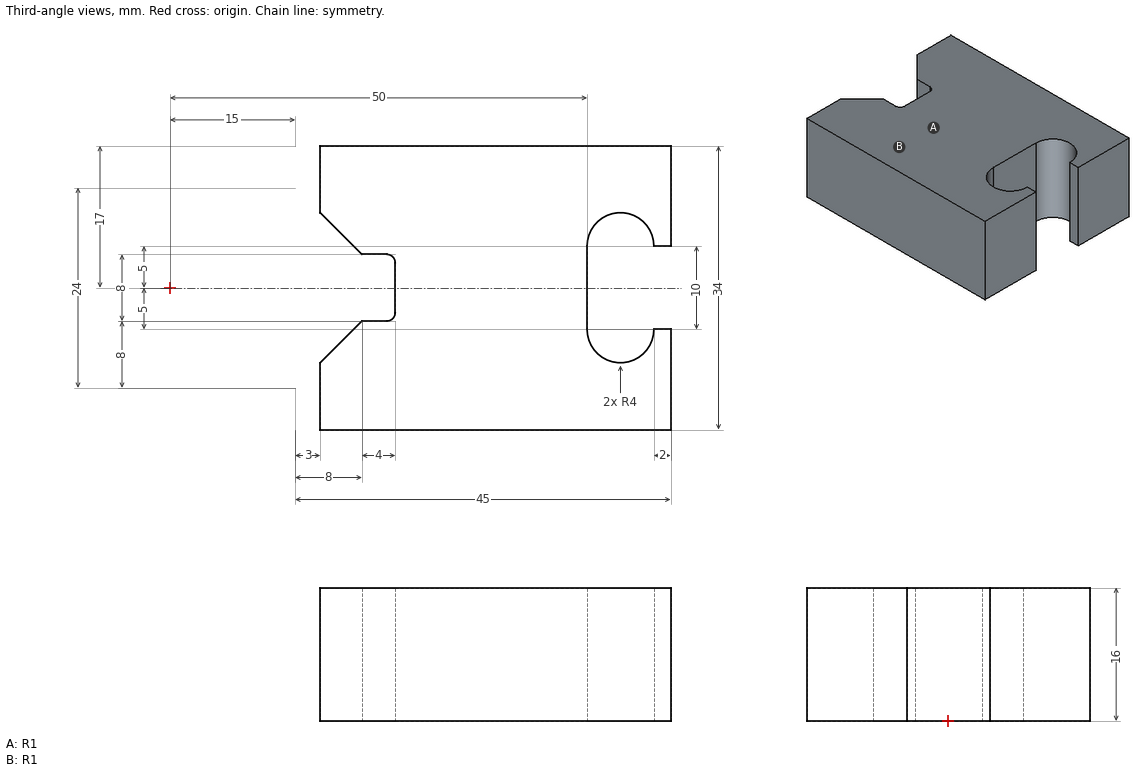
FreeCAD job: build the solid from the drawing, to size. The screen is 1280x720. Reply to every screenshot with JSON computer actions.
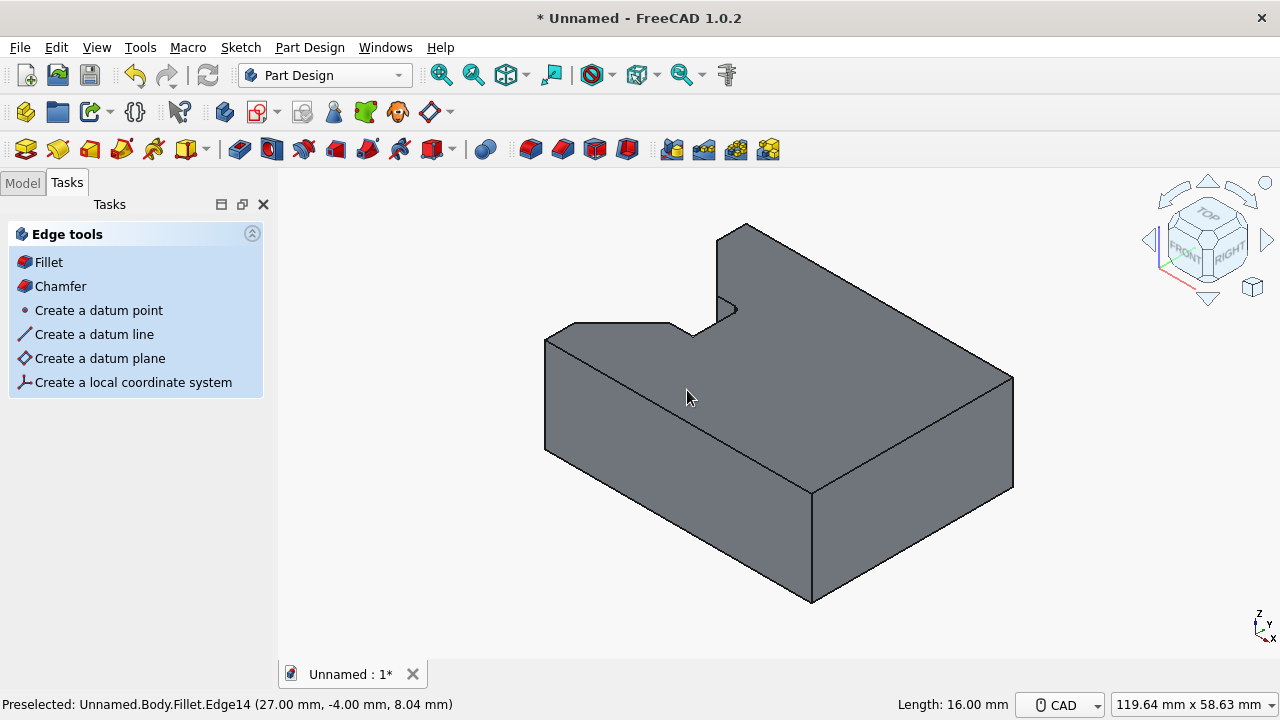
{"action": "left_click", "coordinate": [532, 150]}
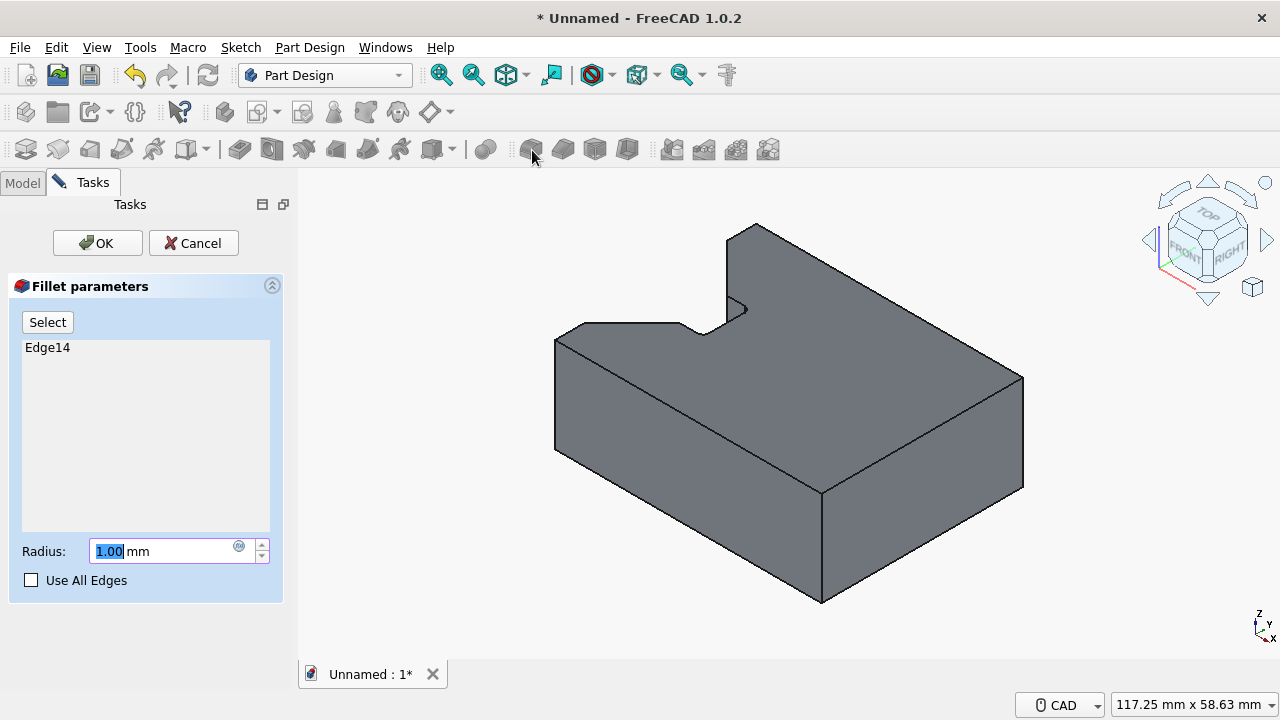
{"action": "type", "text": "1"}
{"action": "key", "text": "Tab"}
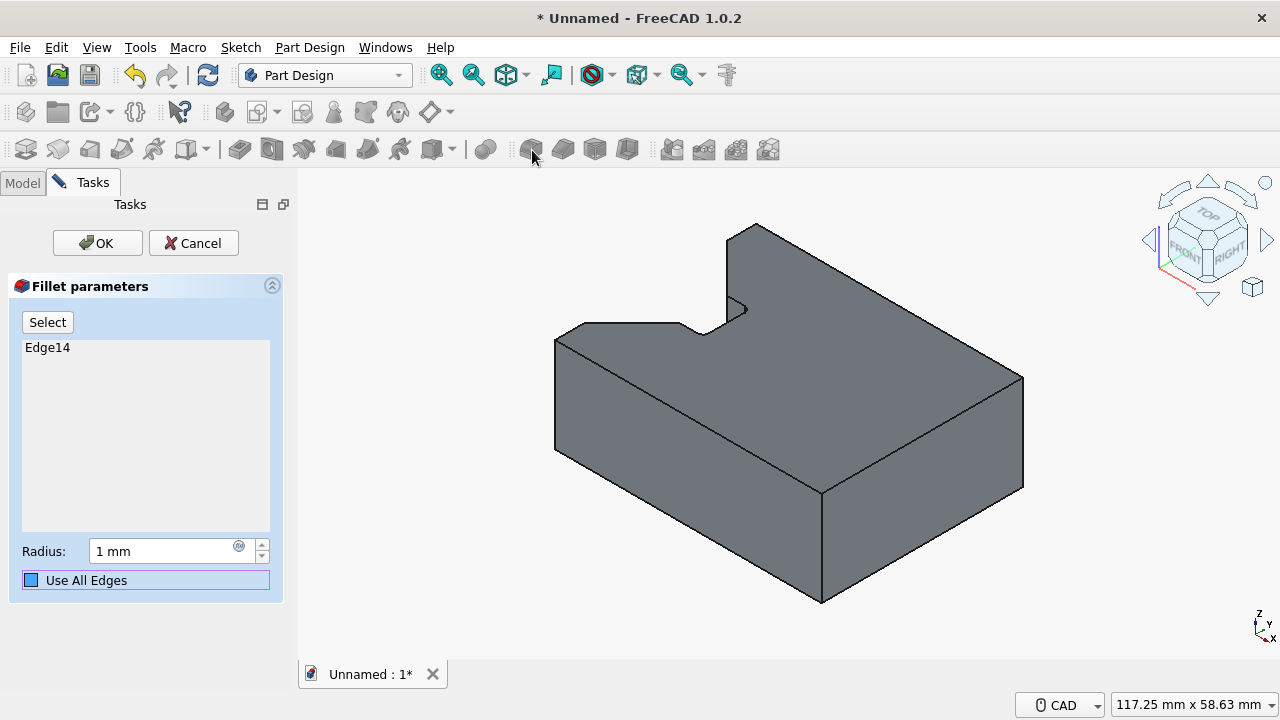
{"action": "left_click", "coordinate": [98, 243]}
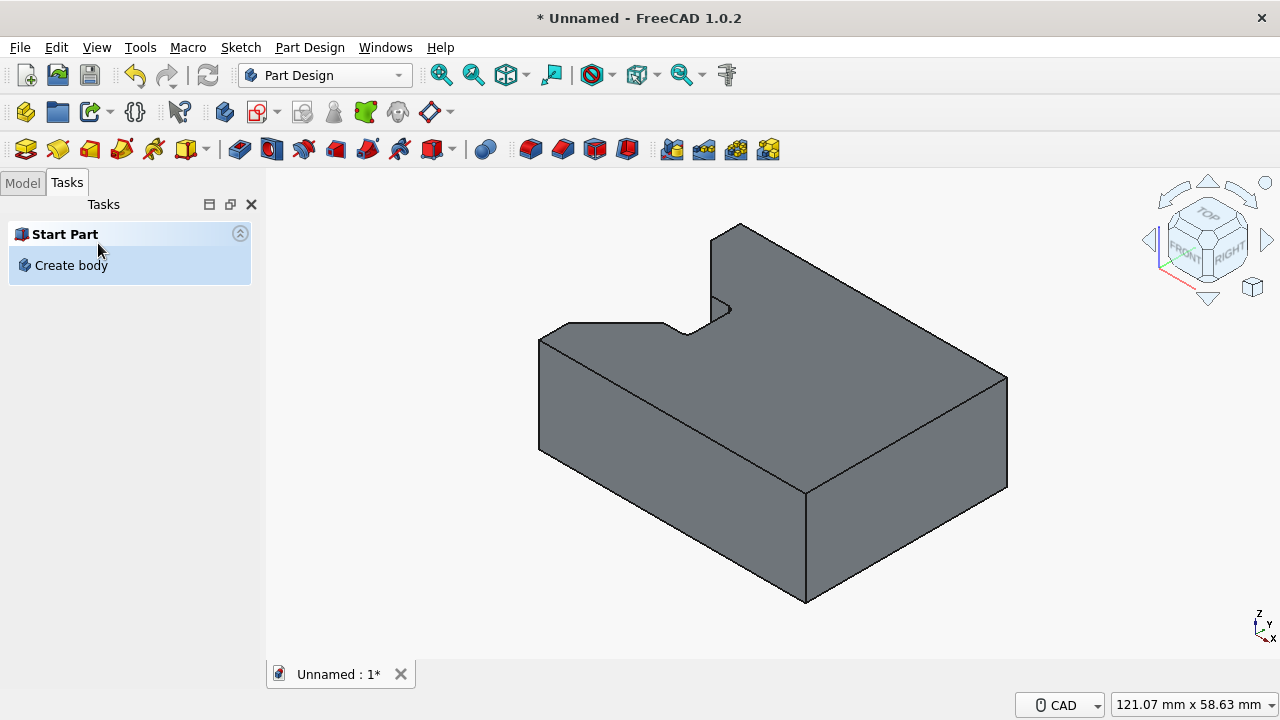
{"action": "left_click", "coordinate": [811, 380]}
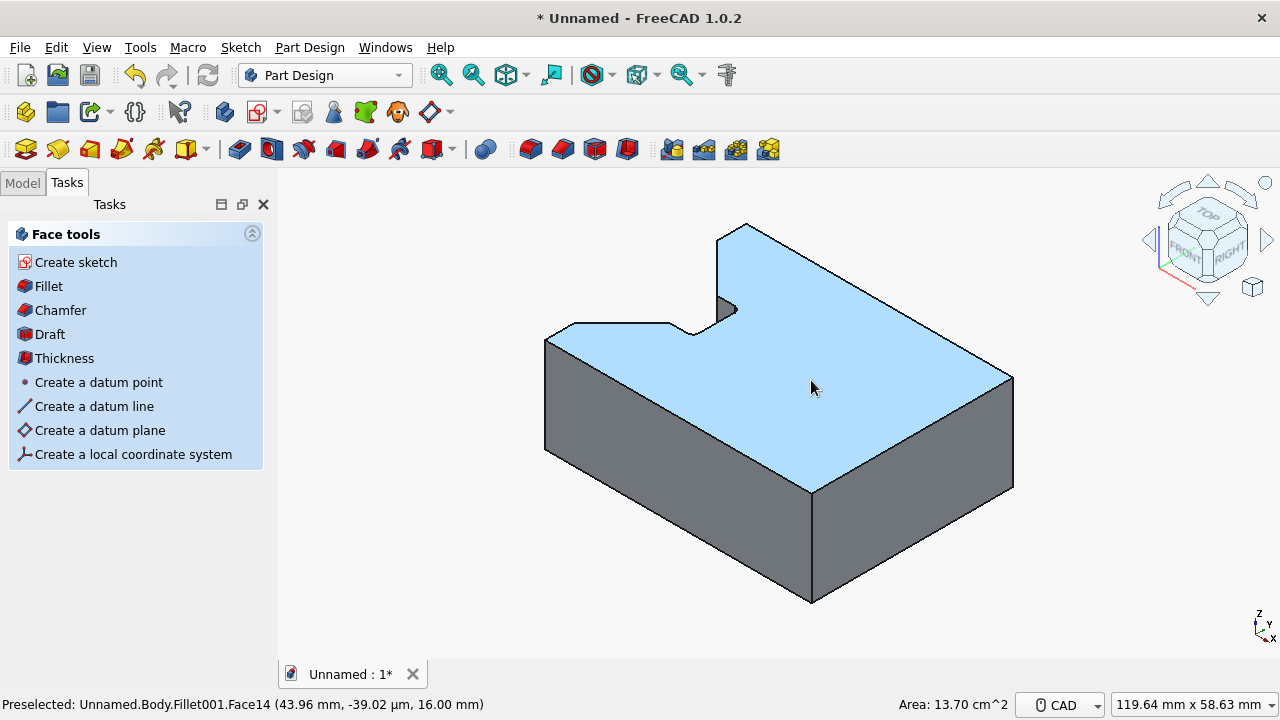
{"action": "left_click", "coordinate": [258, 112]}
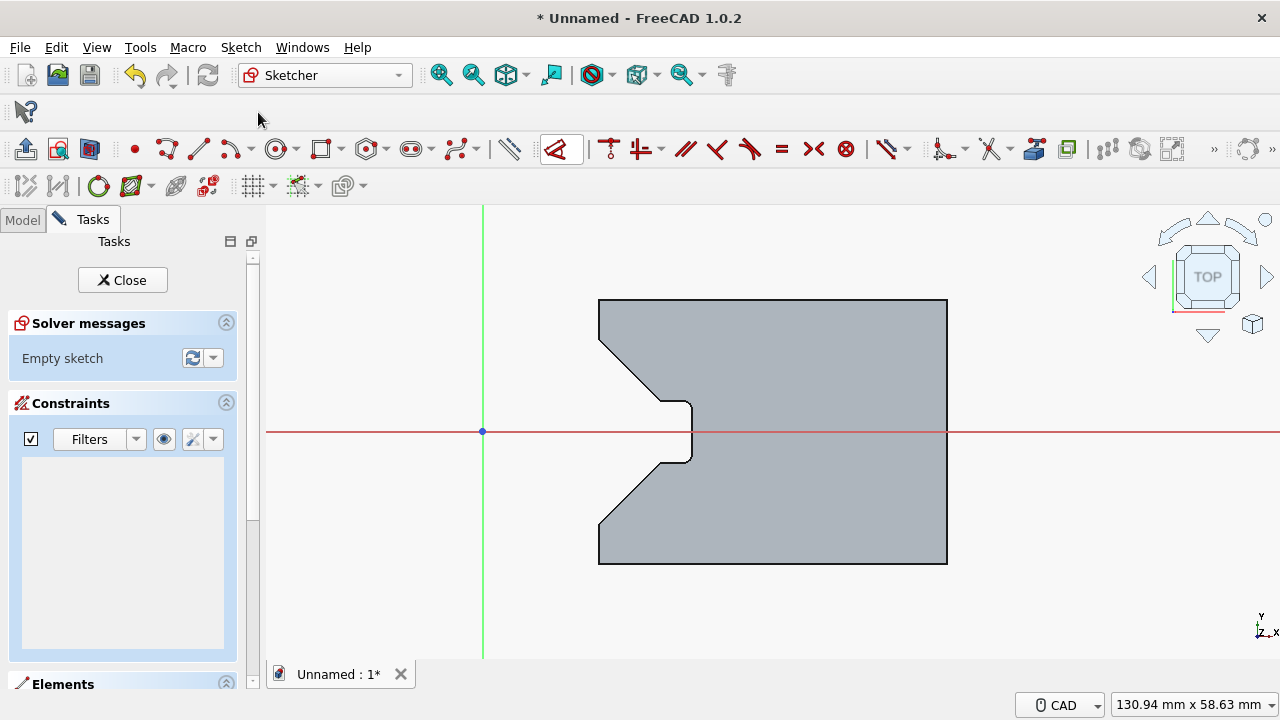
{"action": "scroll", "coordinate": [1075, 432], "scroll_direction": "up", "scroll_amount": 4}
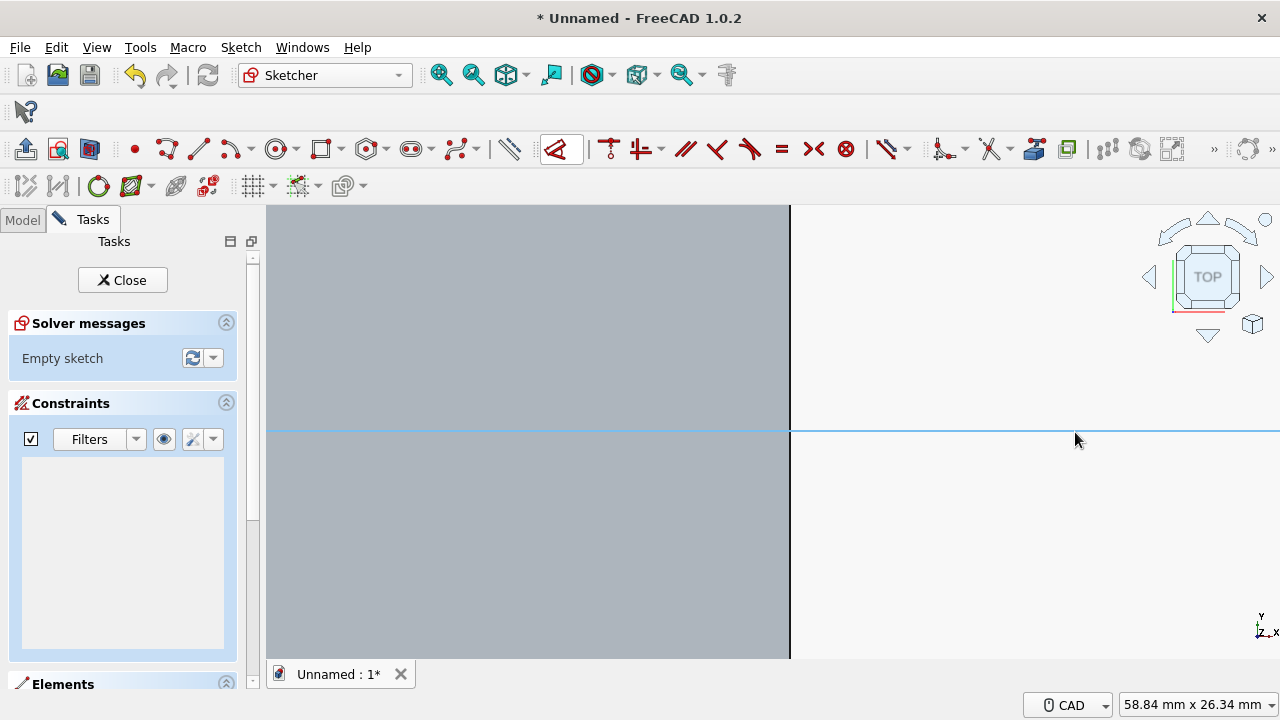
{"action": "left_click", "coordinate": [200, 150]}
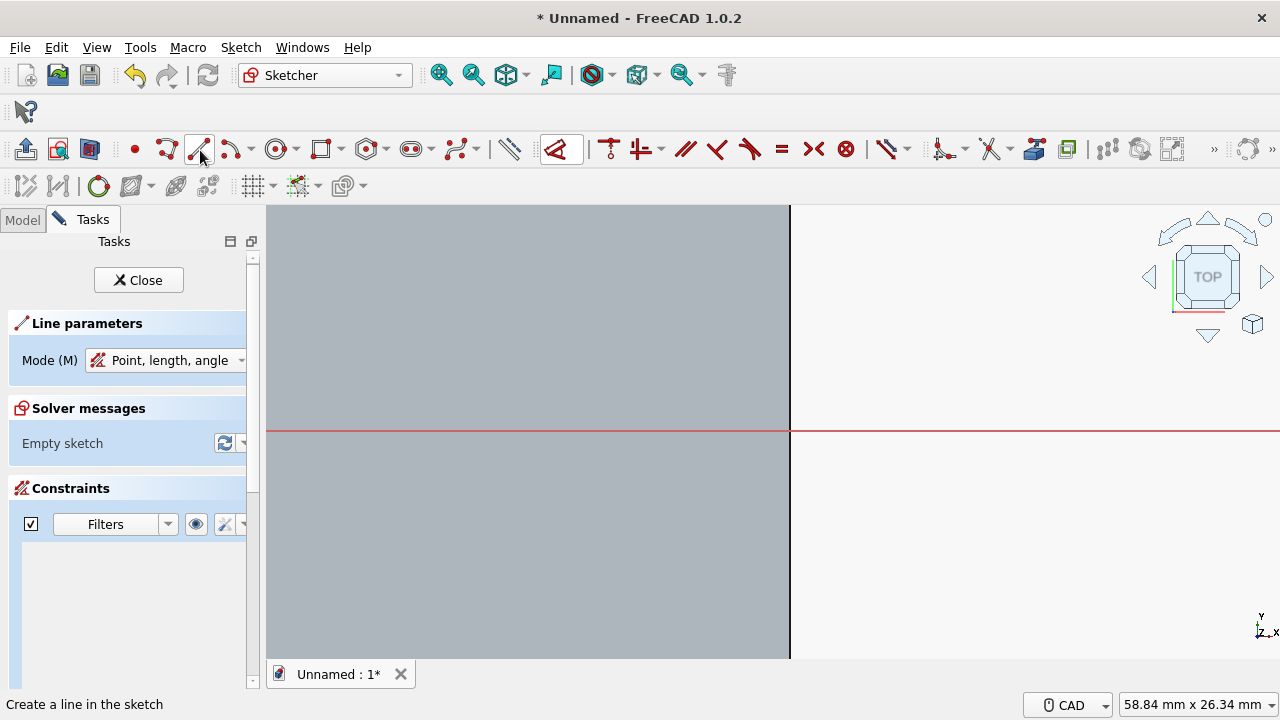
{"action": "left_click", "coordinate": [617, 345]}
{"action": "left_click", "coordinate": [617, 518]}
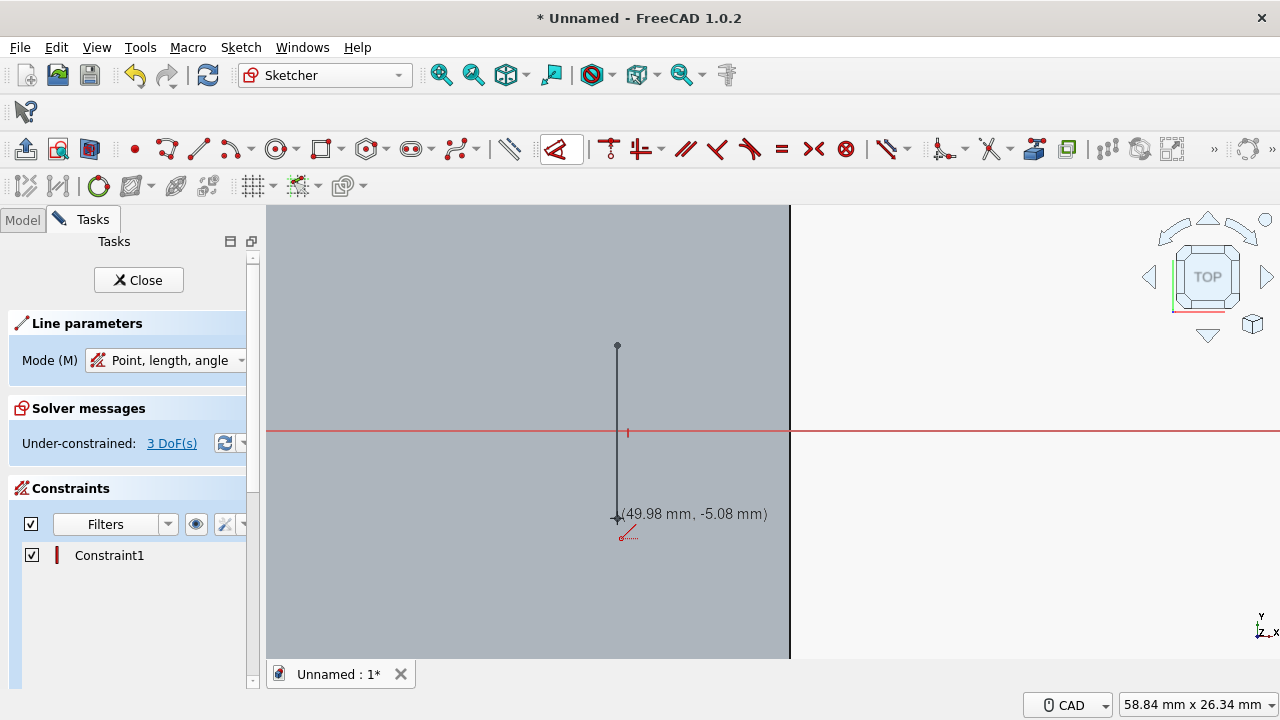
{"action": "left_click", "coordinate": [168, 150]}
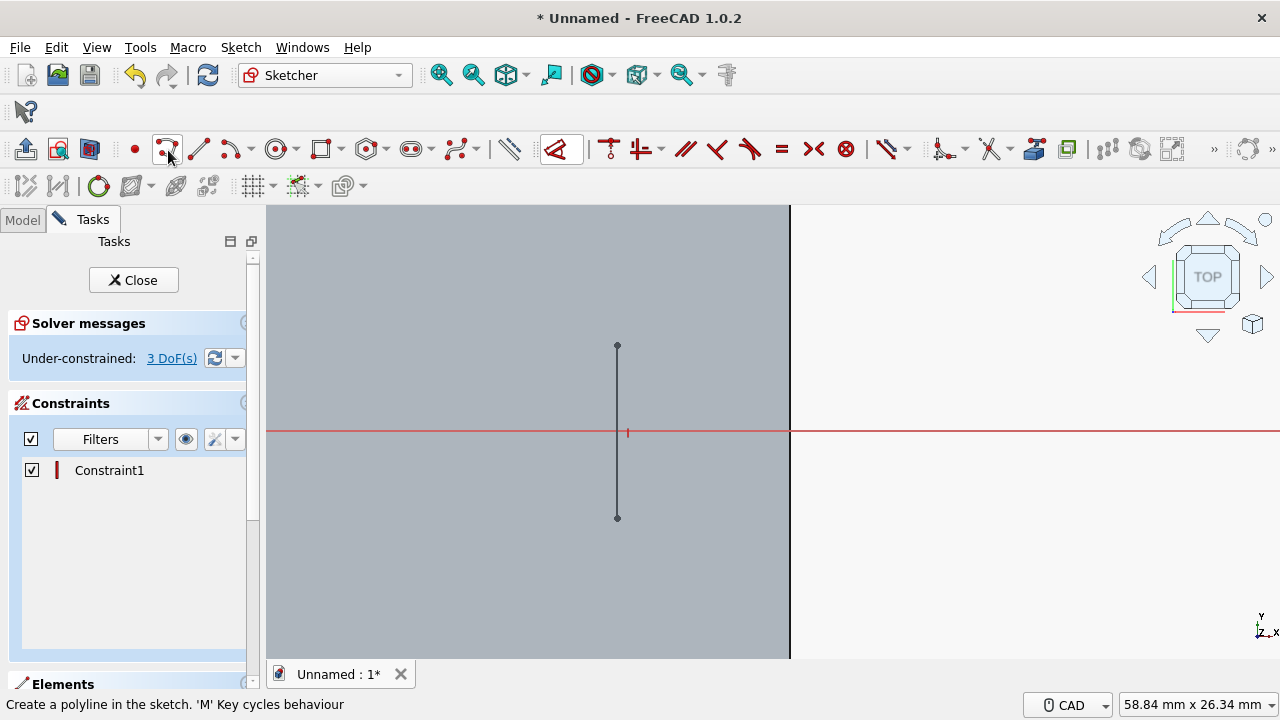
{"action": "left_click", "coordinate": [755, 518]}
{"action": "left_click", "coordinate": [790, 518]}
{"action": "left_click", "coordinate": [790, 345]}
{"action": "left_click", "coordinate": [755, 345]}
{"action": "right_click", "coordinate": [755, 345]}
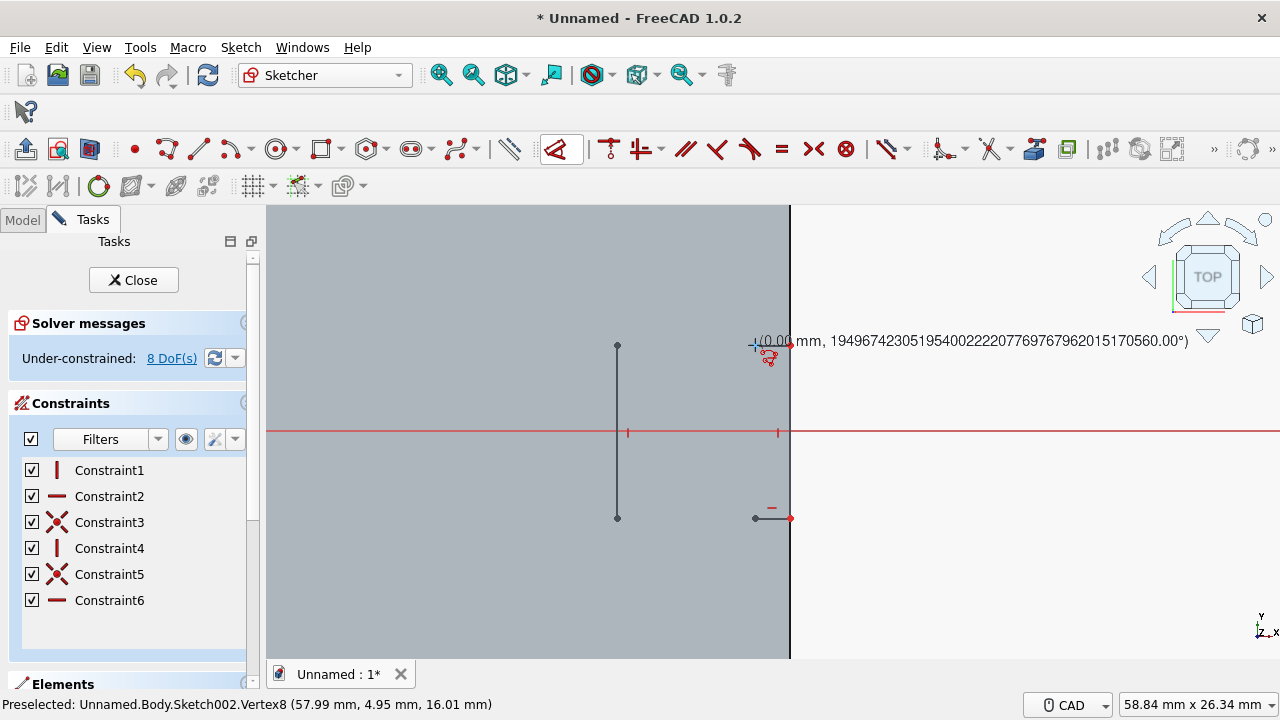
{"action": "left_click", "coordinate": [254, 150]}